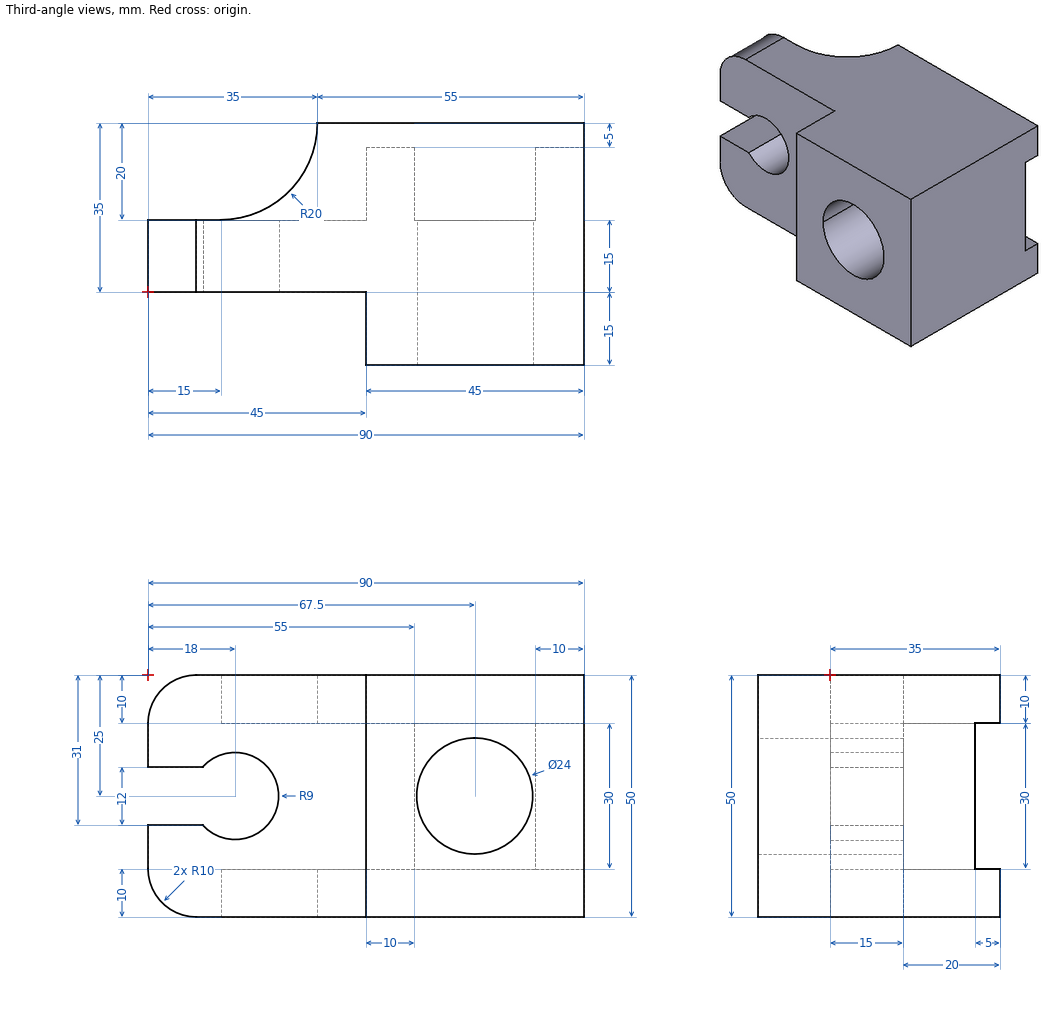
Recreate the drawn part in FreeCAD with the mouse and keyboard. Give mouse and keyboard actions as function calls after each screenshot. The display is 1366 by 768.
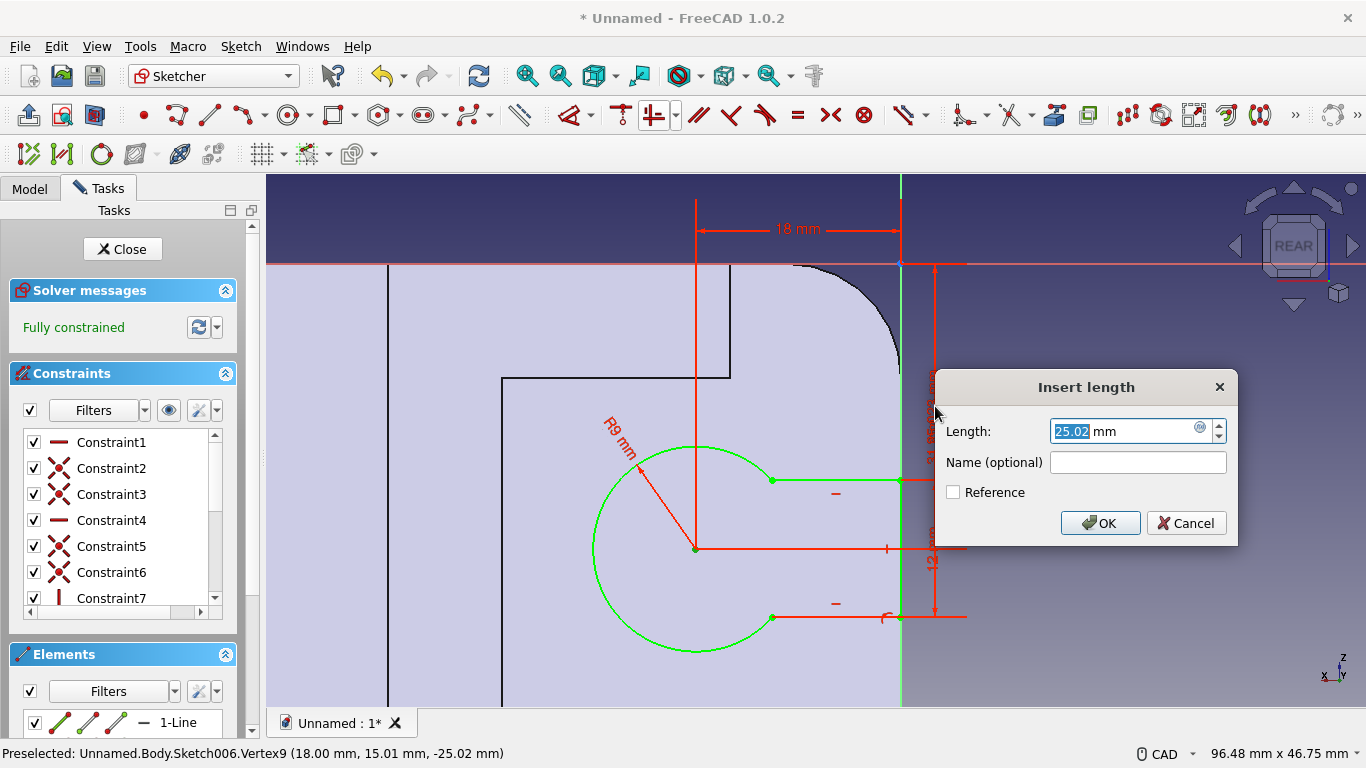
text(25)
key(Return)
key(Escape)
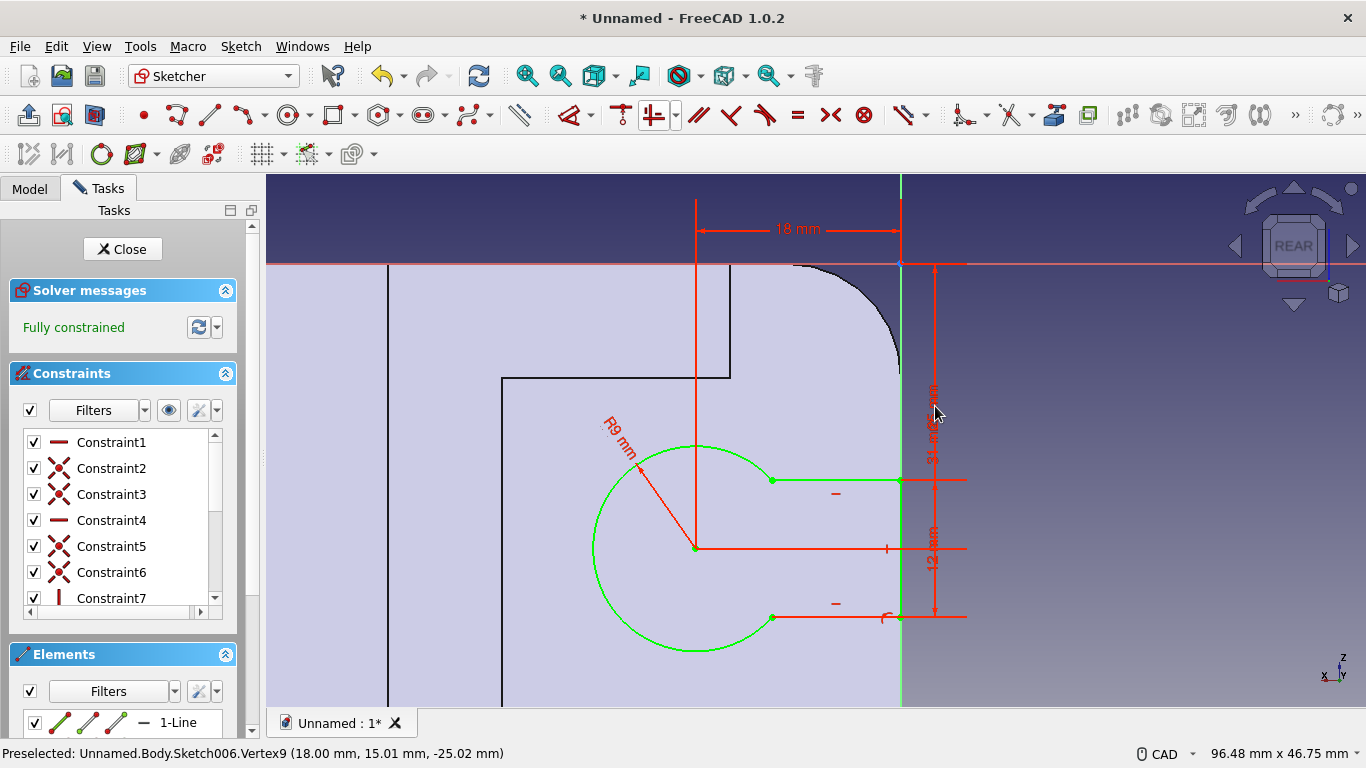
click(123, 249)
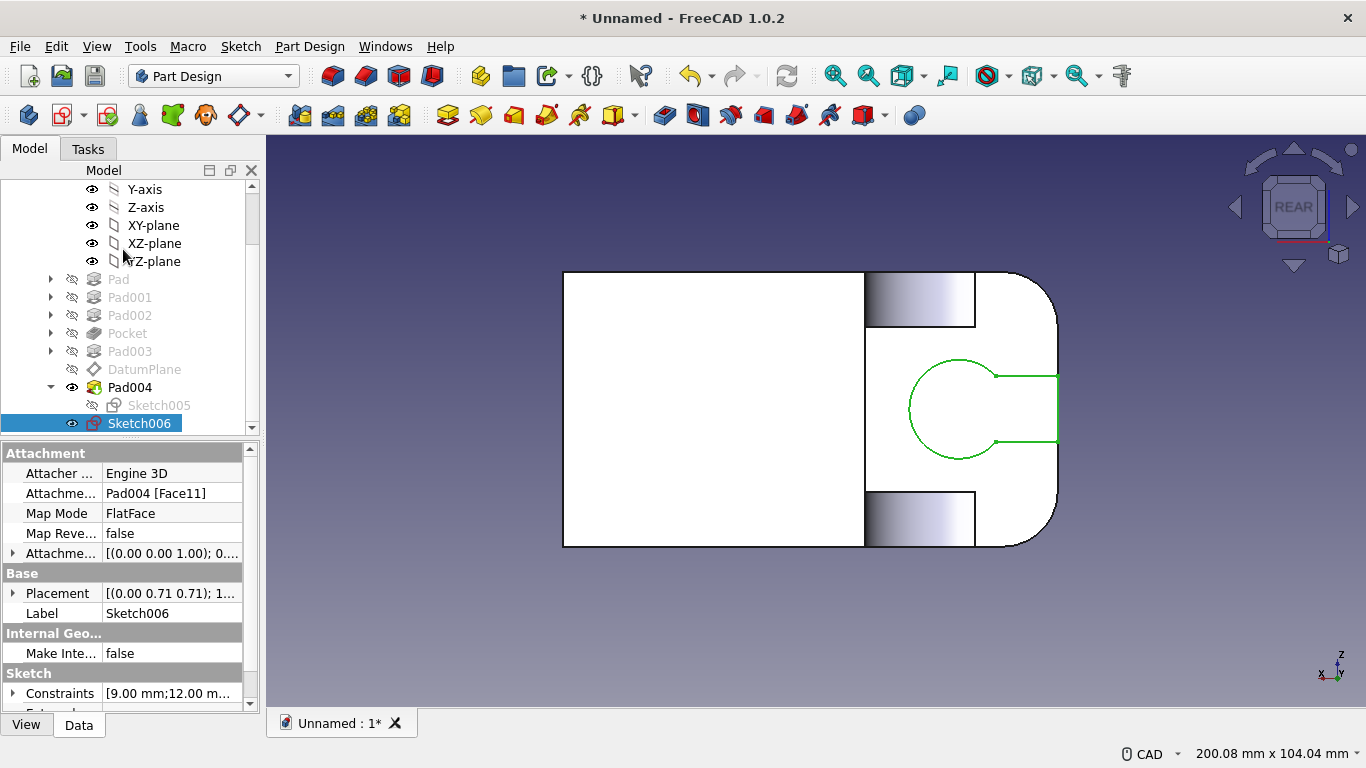
click(665, 116)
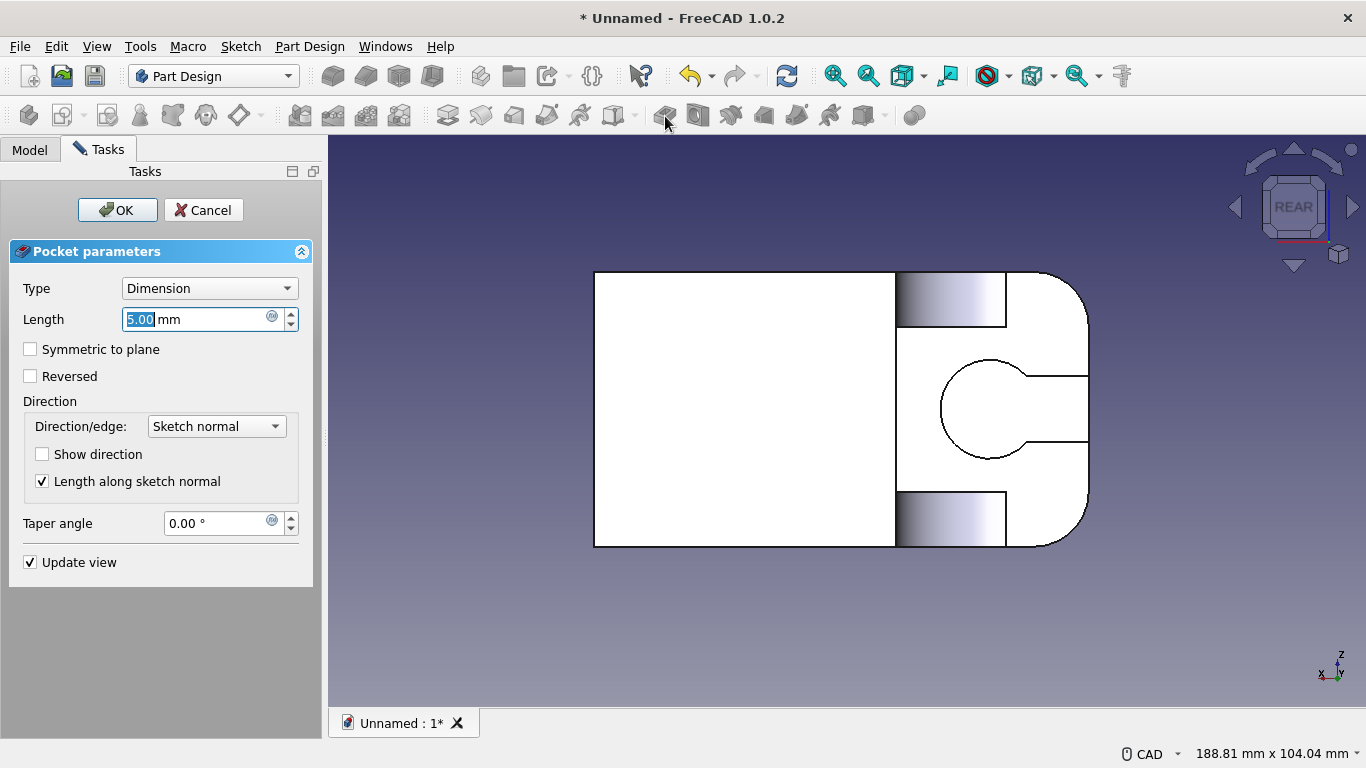
text(15)
key(Tab)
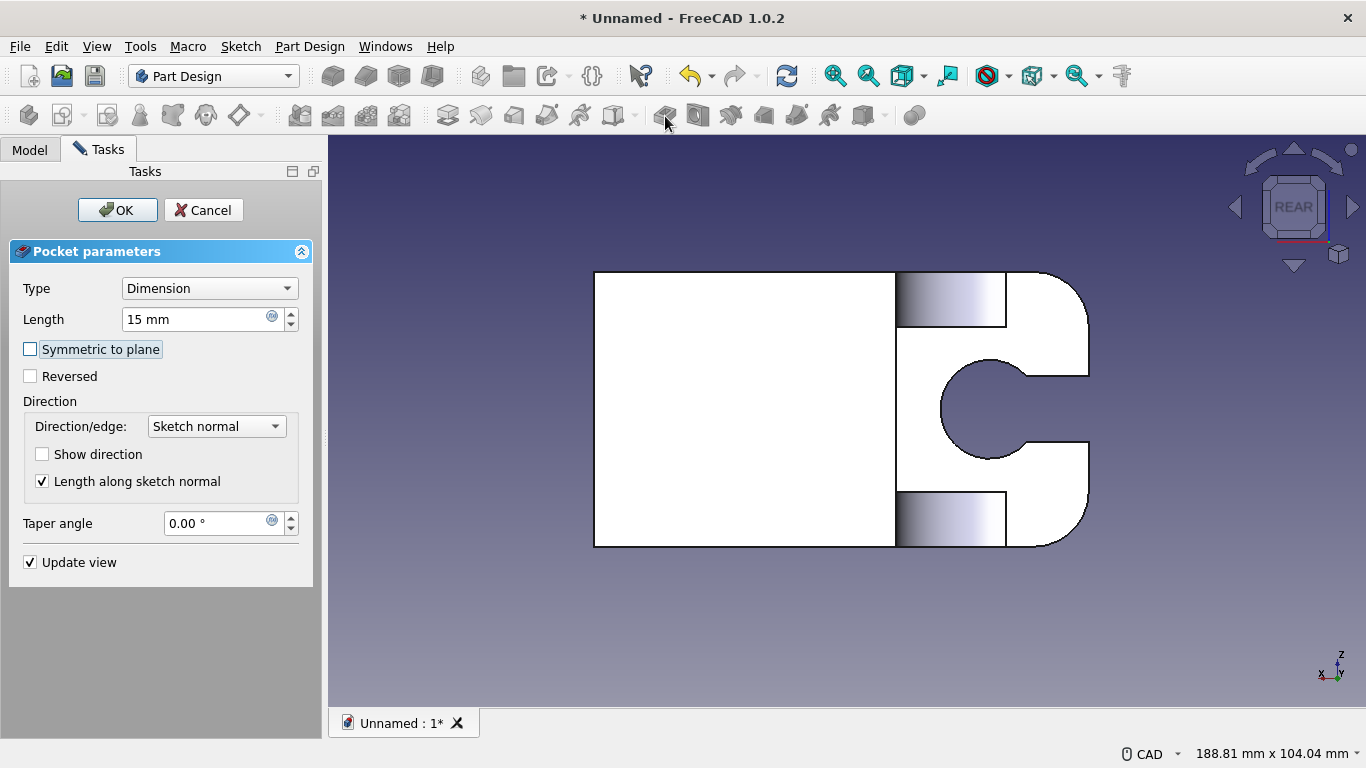
click(118, 210)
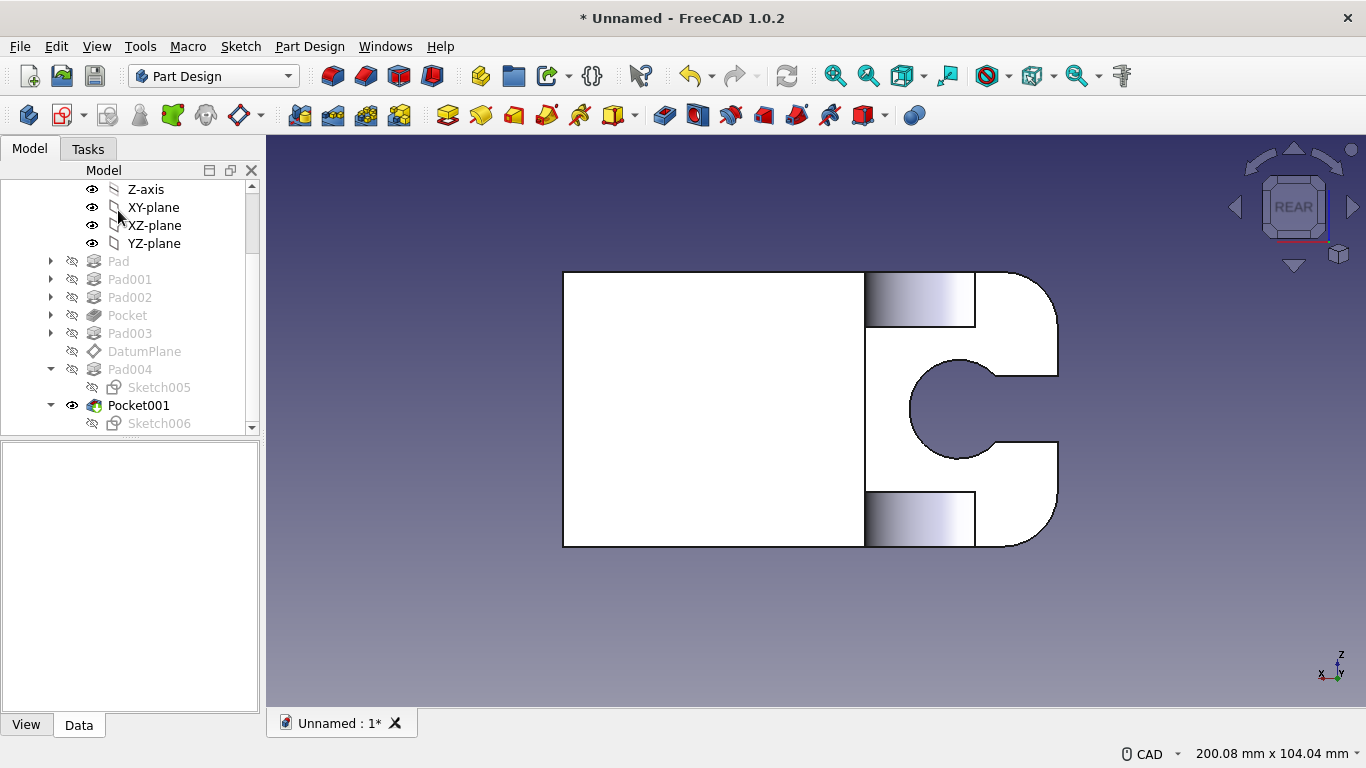
key(6)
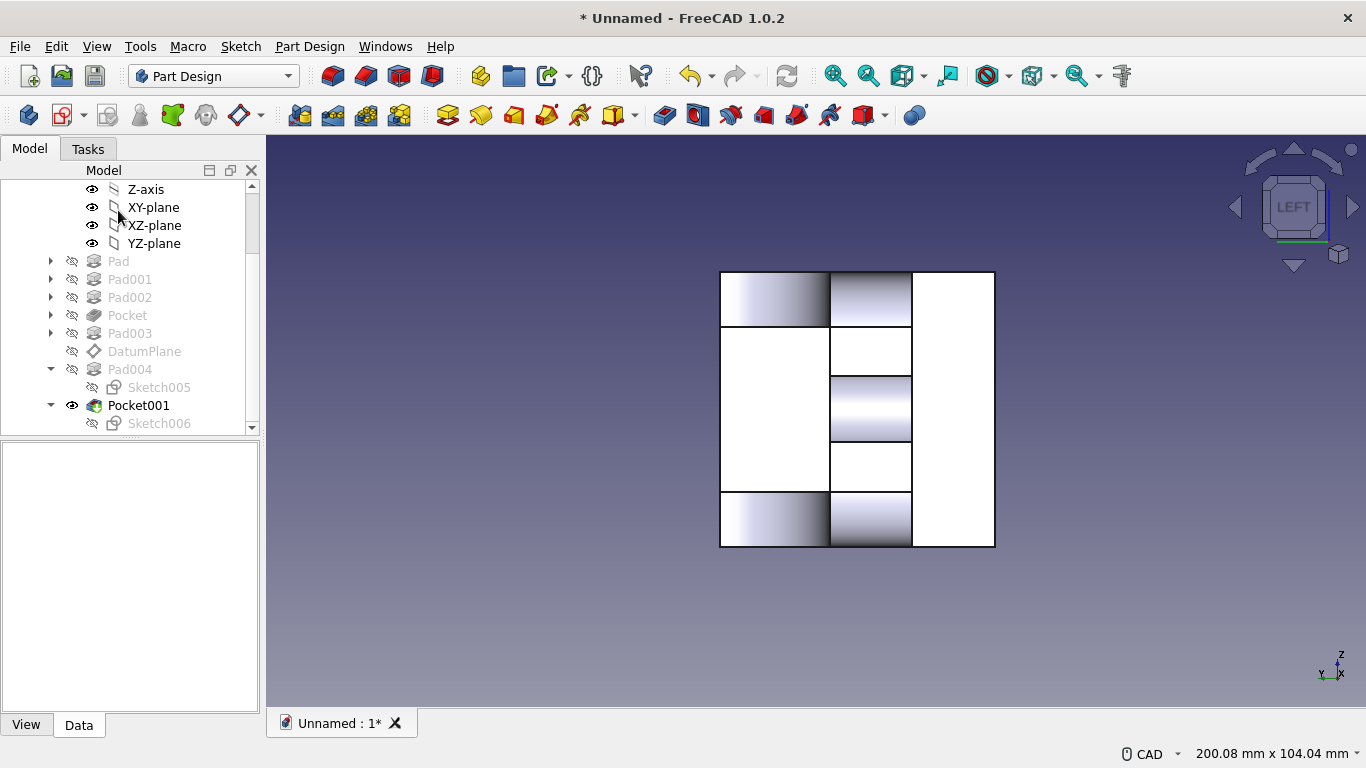
click(775, 385)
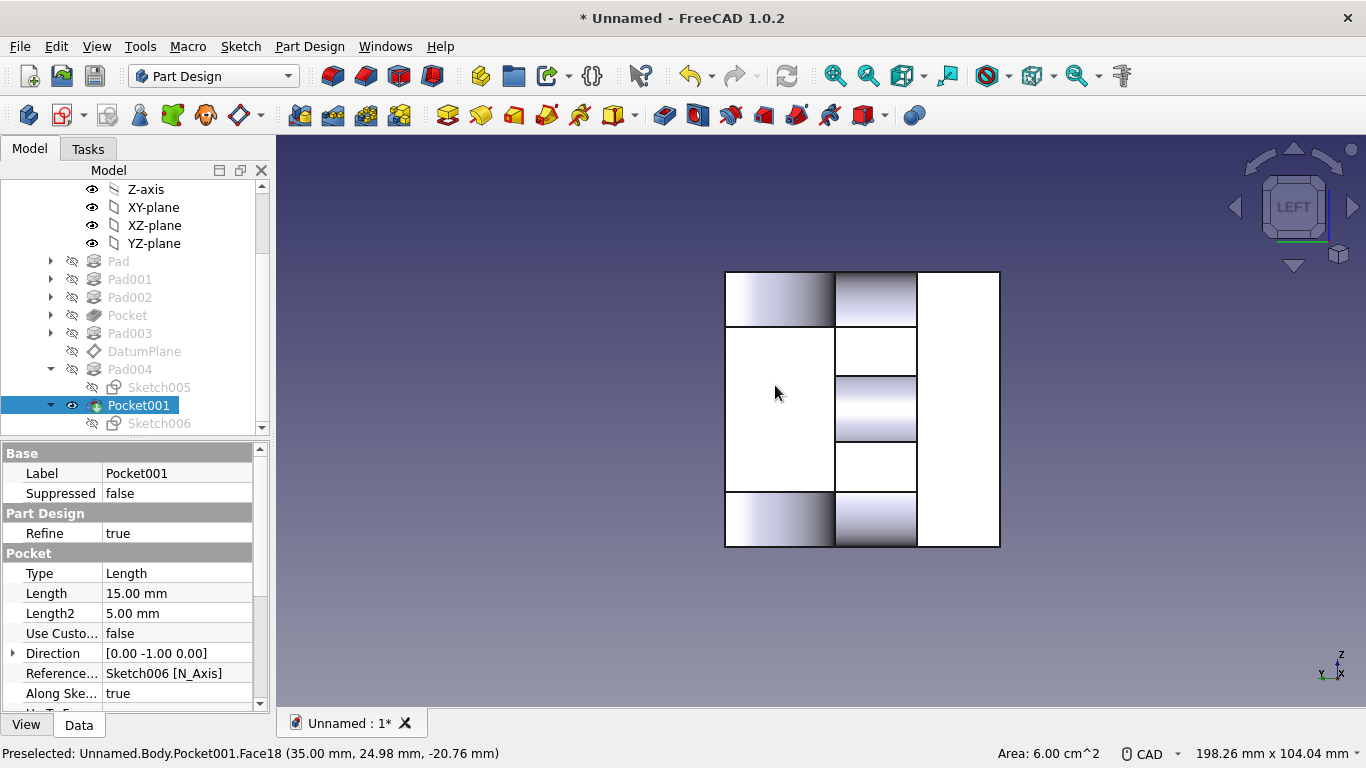
click(62, 116)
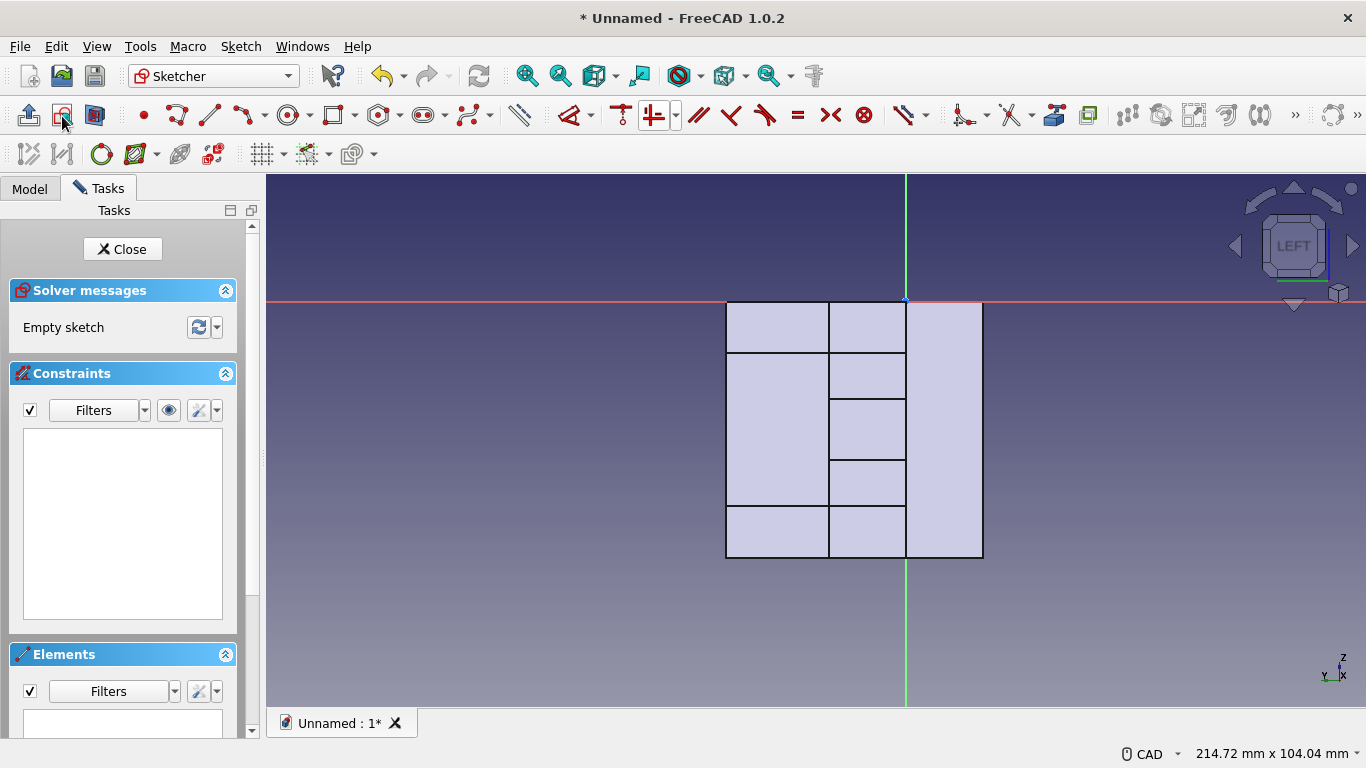
click(95, 116)